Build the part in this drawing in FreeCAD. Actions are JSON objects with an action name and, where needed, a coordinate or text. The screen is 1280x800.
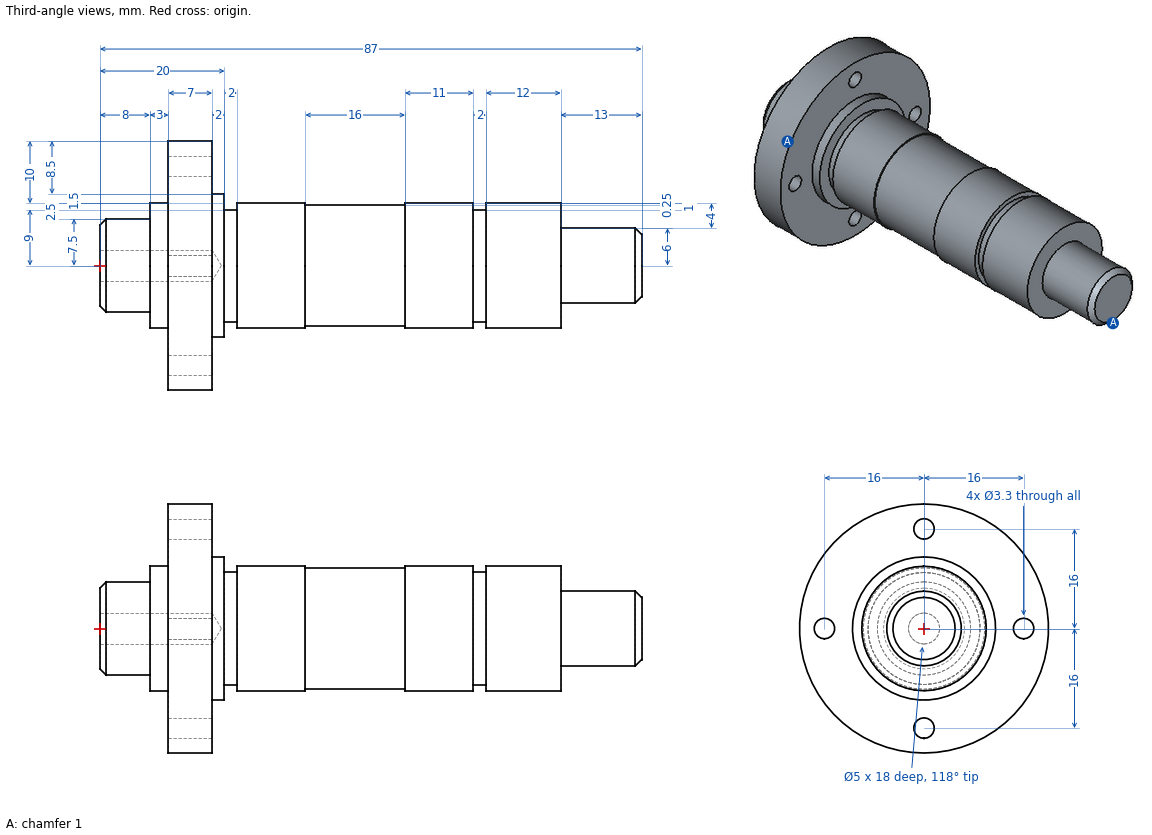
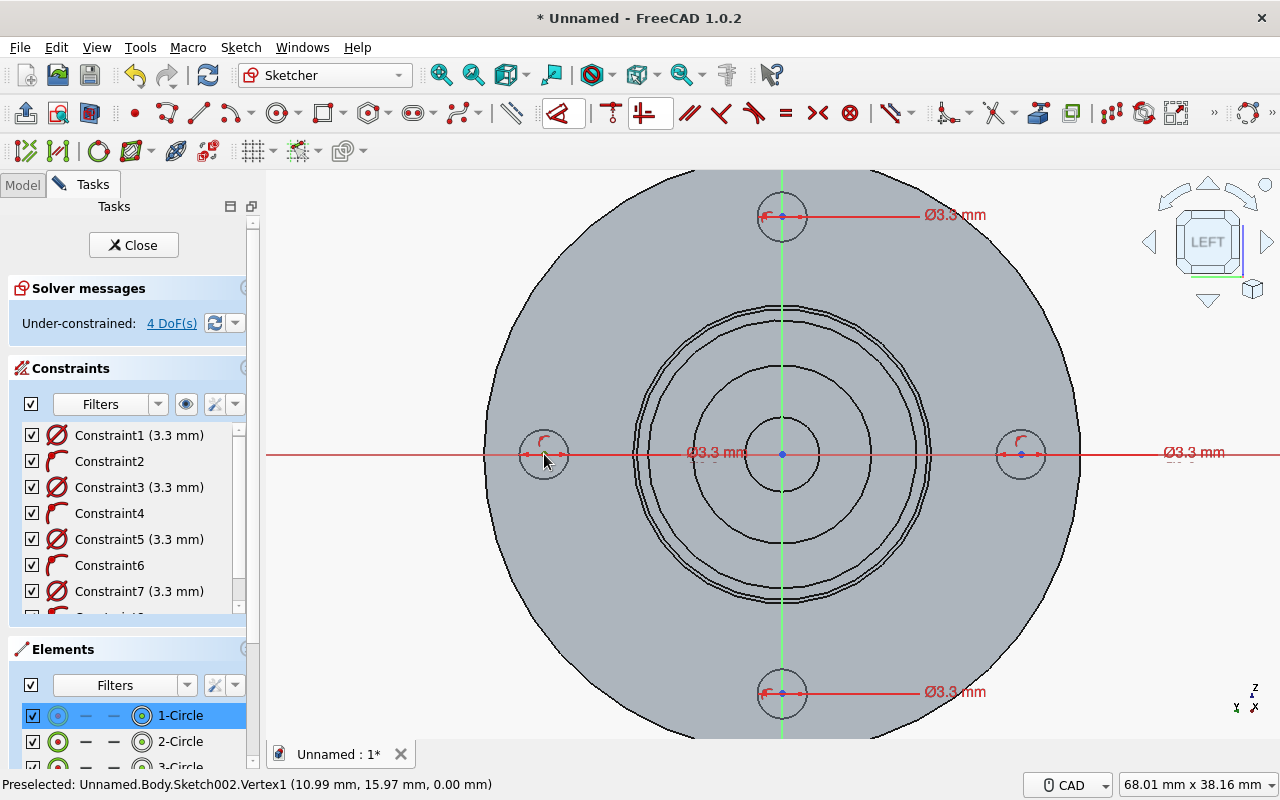
{"action": "left_click", "coordinate": [580, 114]}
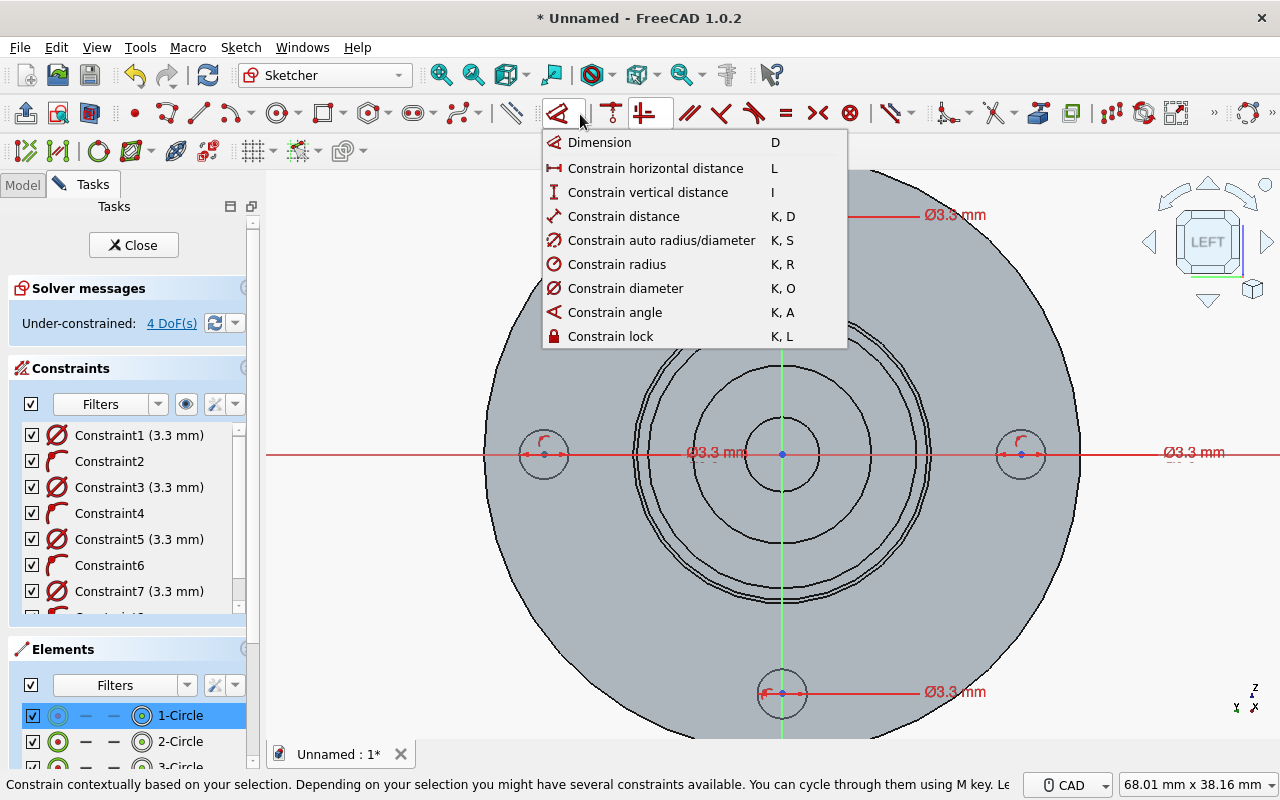
{"action": "left_click", "coordinate": [695, 168]}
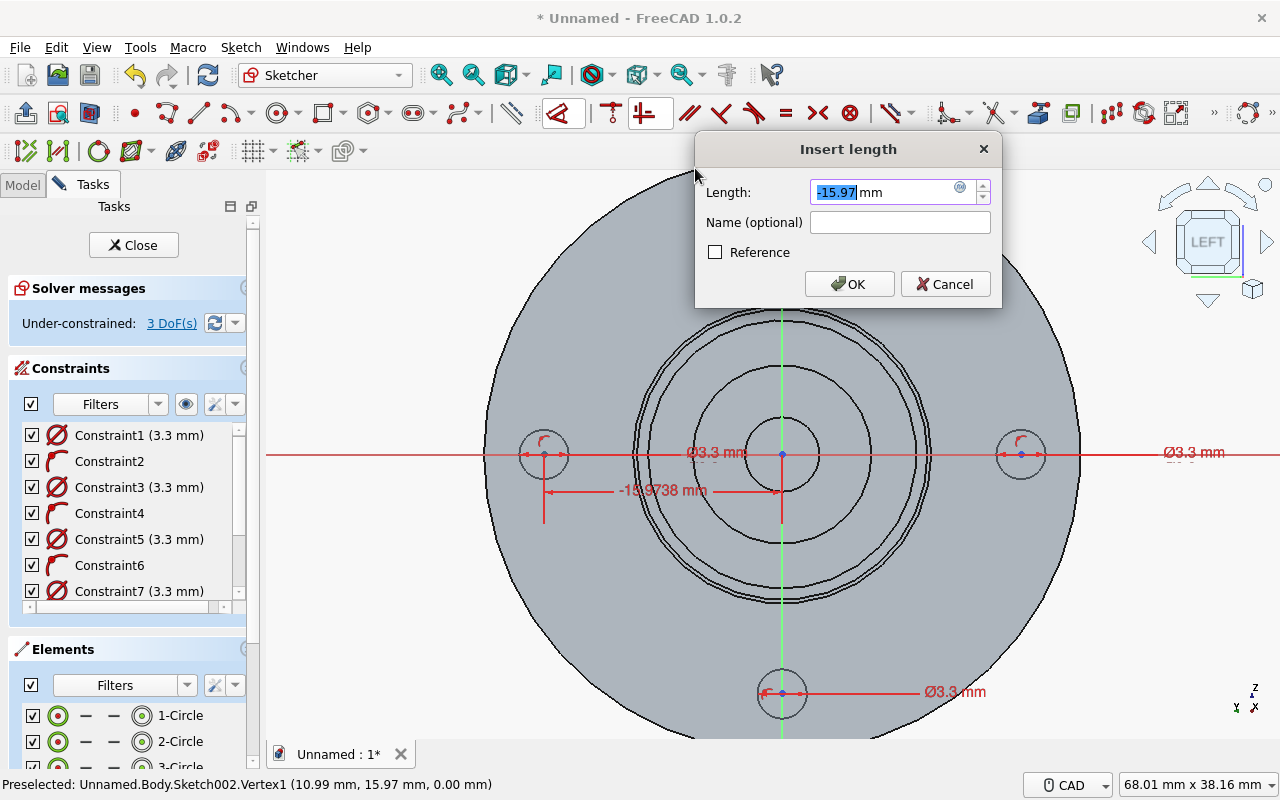
{"action": "type", "text": "-16"}
{"action": "key", "text": "Return"}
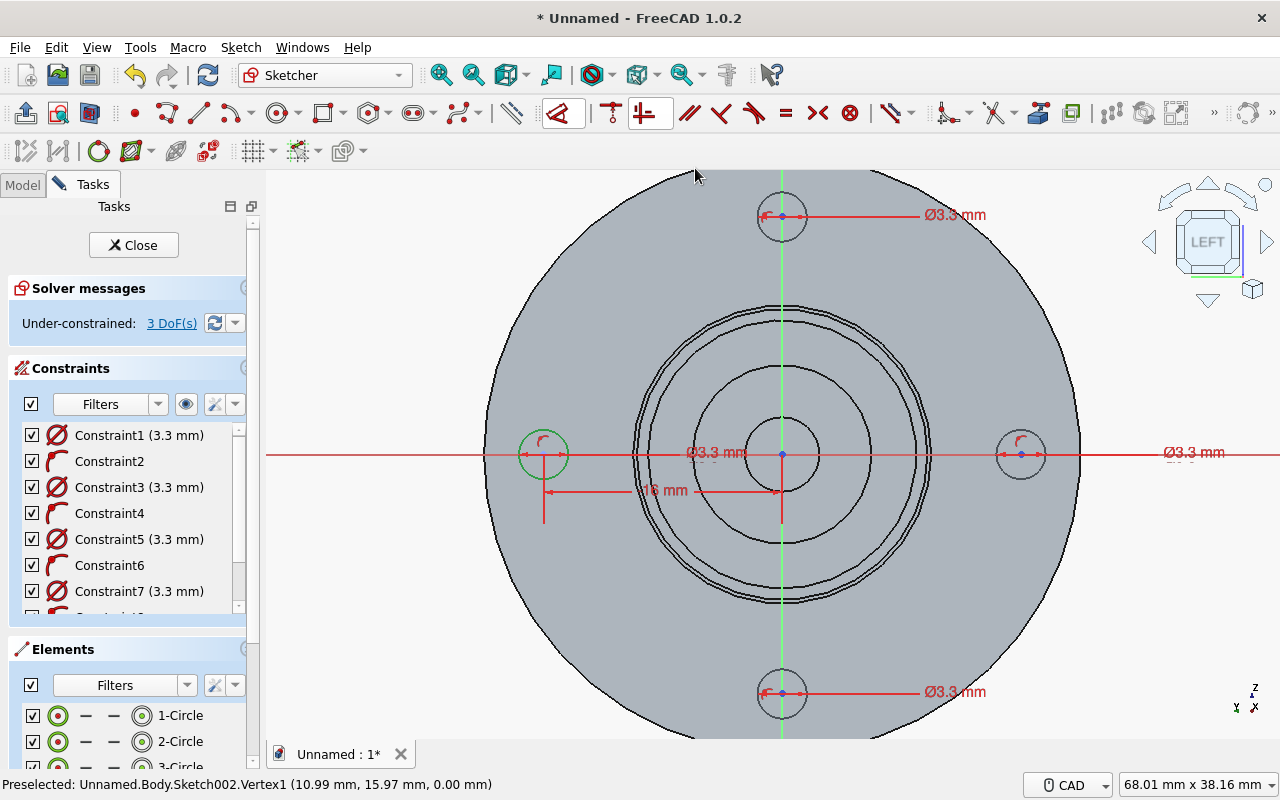
{"action": "left_click", "coordinate": [782, 694]}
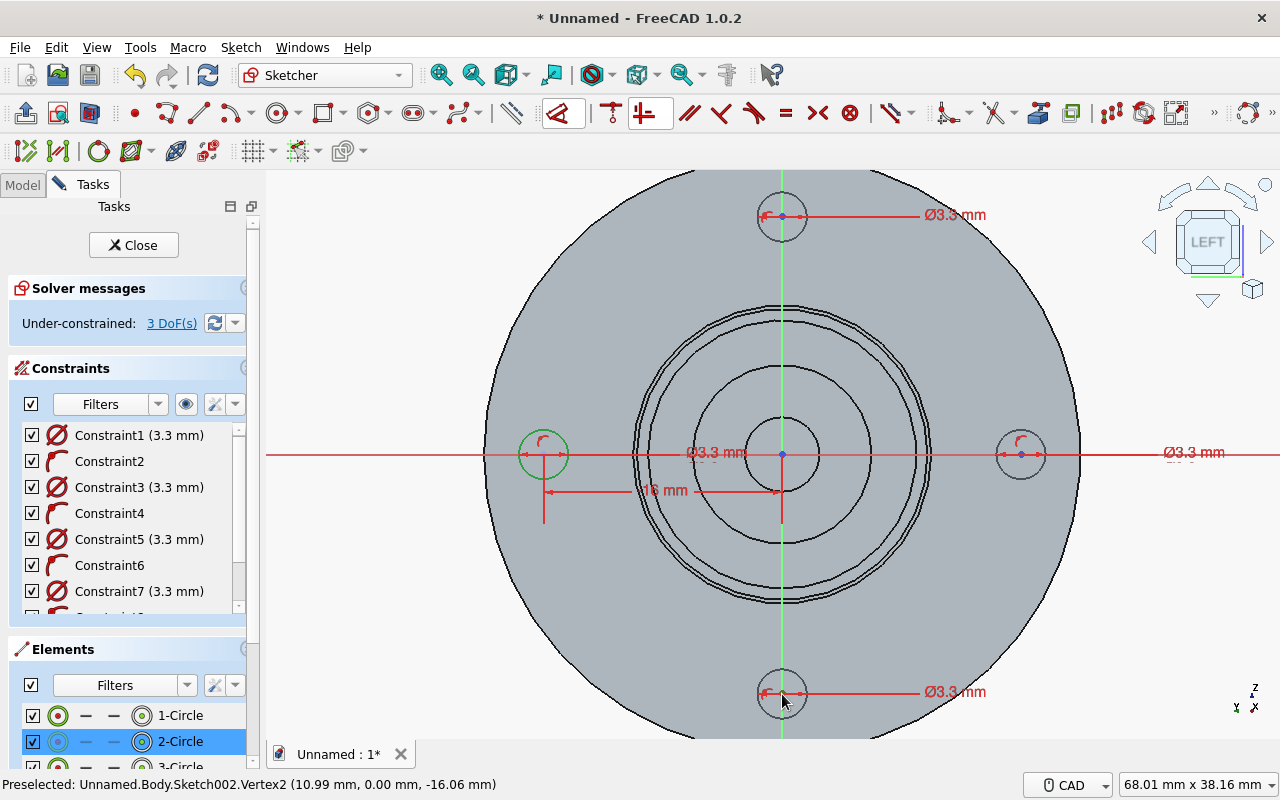
{"action": "left_click", "coordinate": [580, 114]}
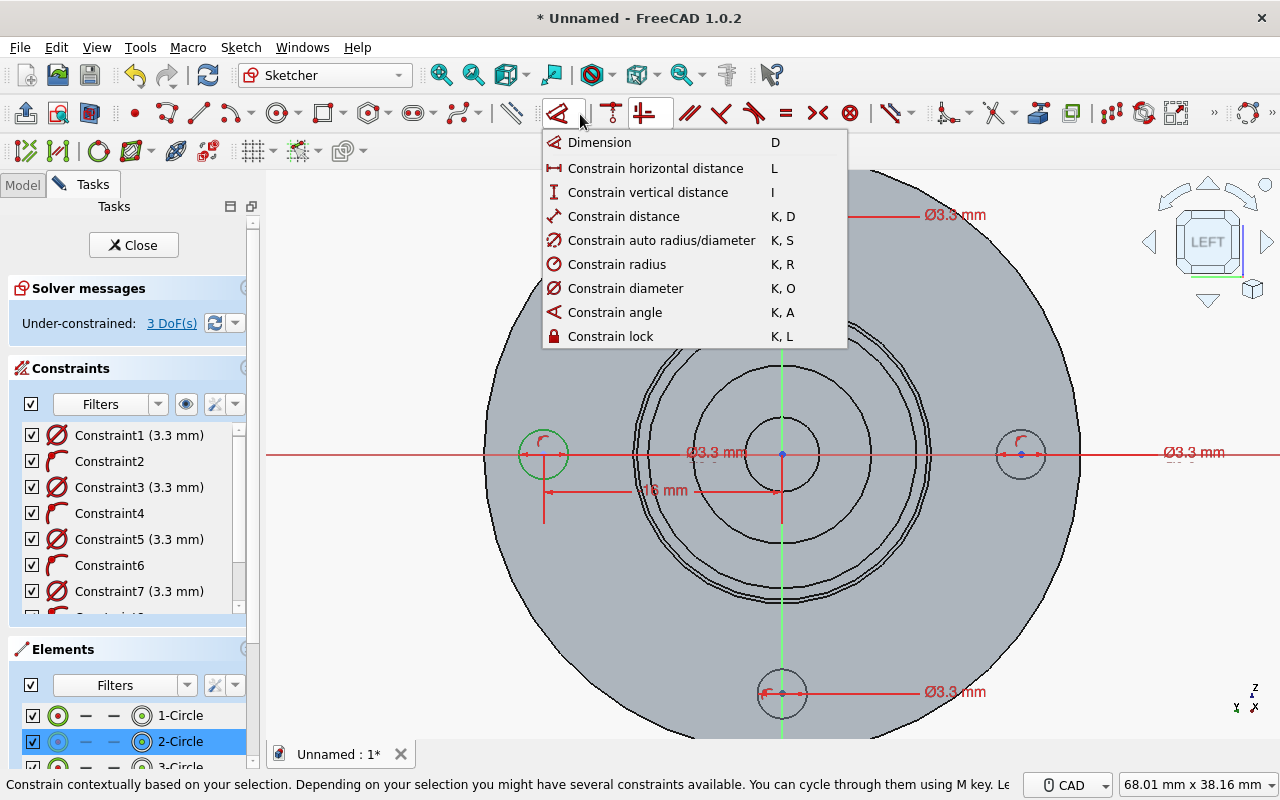
{"action": "left_click", "coordinate": [695, 192]}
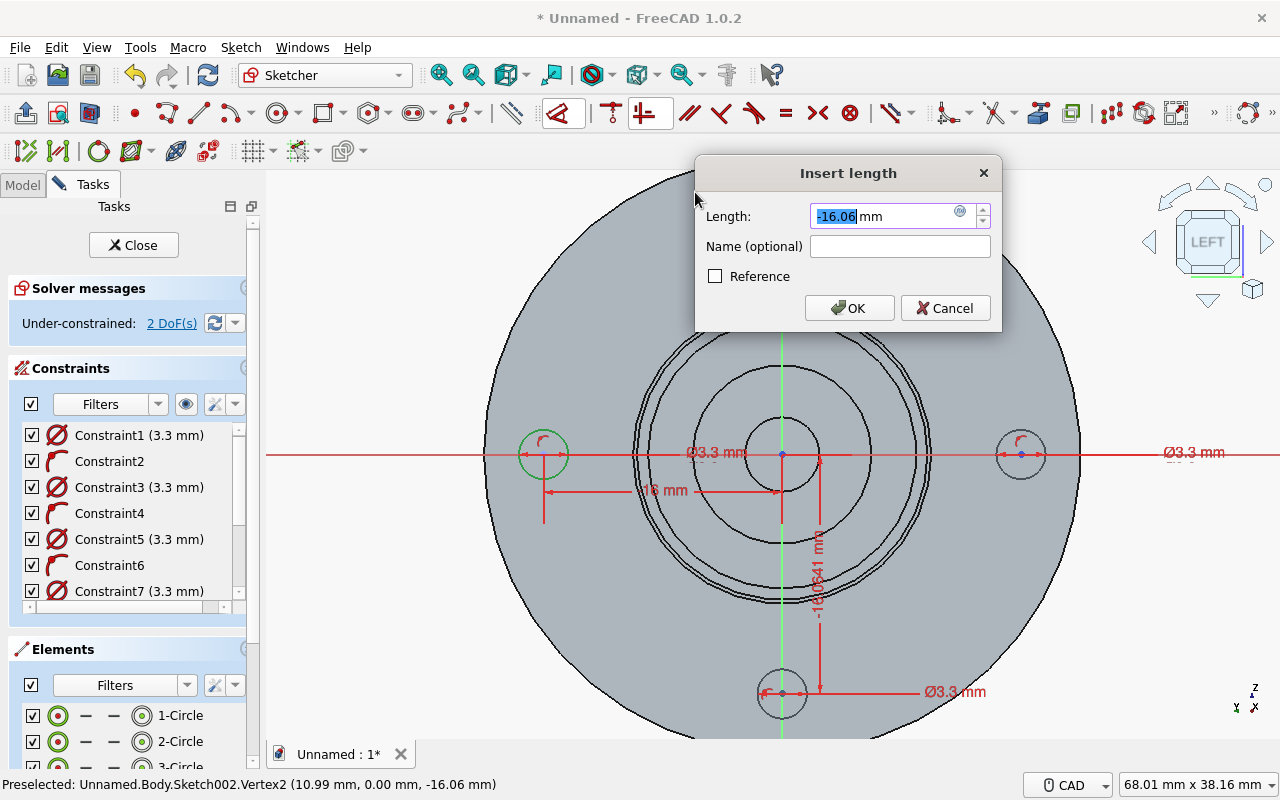
{"action": "type", "text": "-16"}
{"action": "key", "text": "Return"}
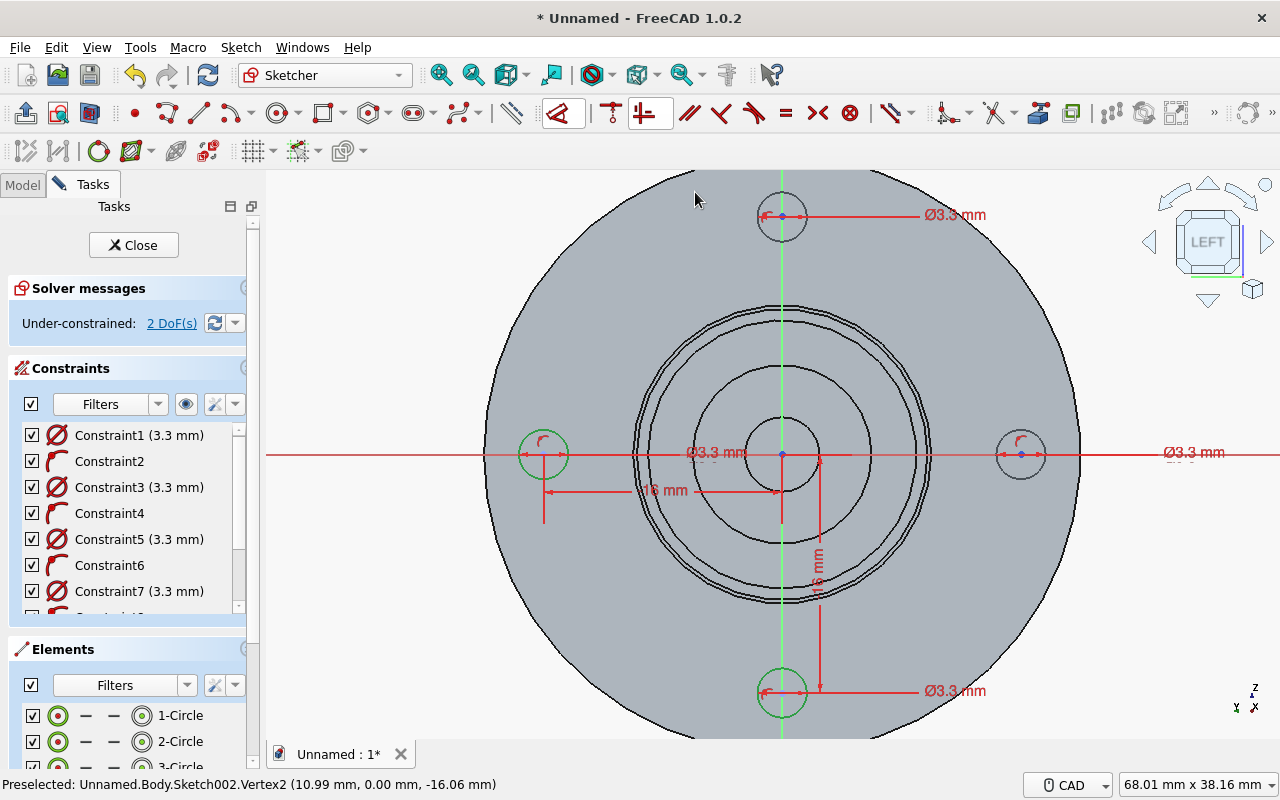
{"action": "left_click", "coordinate": [1021, 454]}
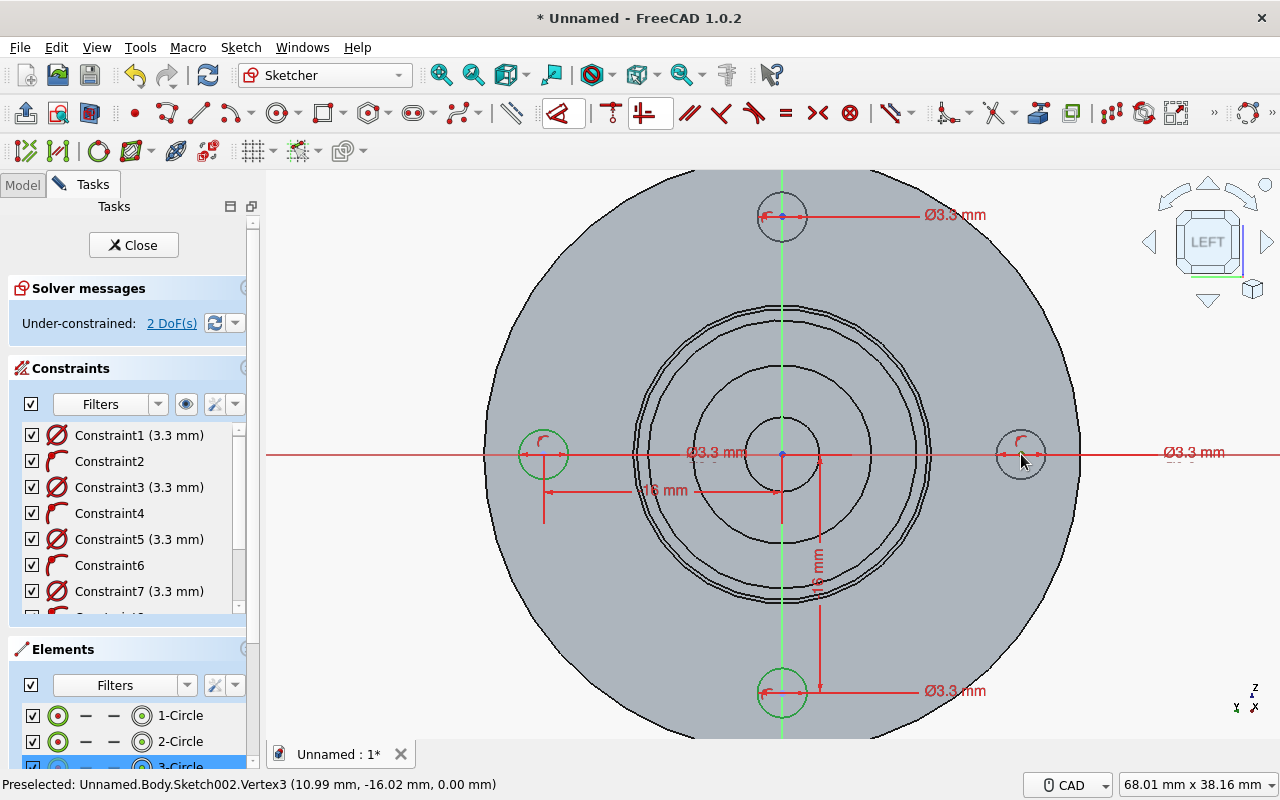
{"action": "key", "text": "l"}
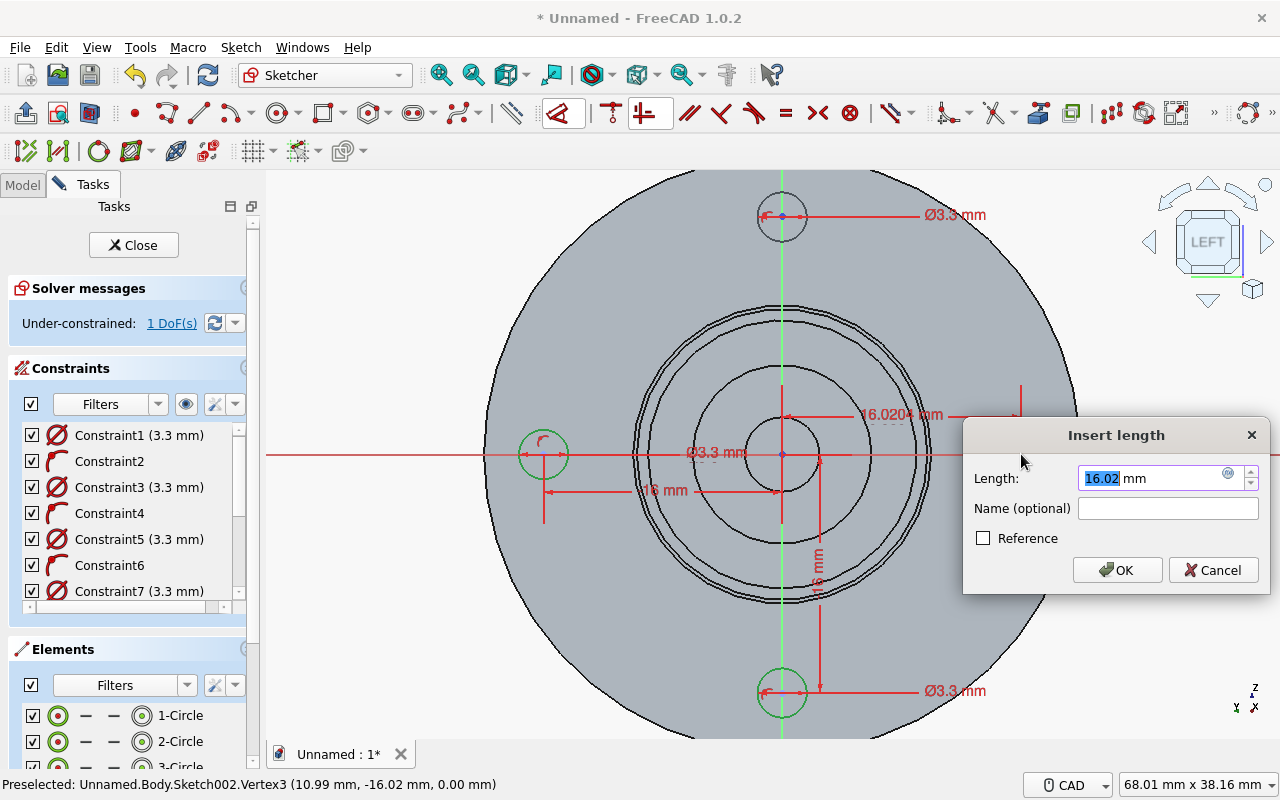
{"action": "type", "text": "16"}
{"action": "key", "text": "Return"}